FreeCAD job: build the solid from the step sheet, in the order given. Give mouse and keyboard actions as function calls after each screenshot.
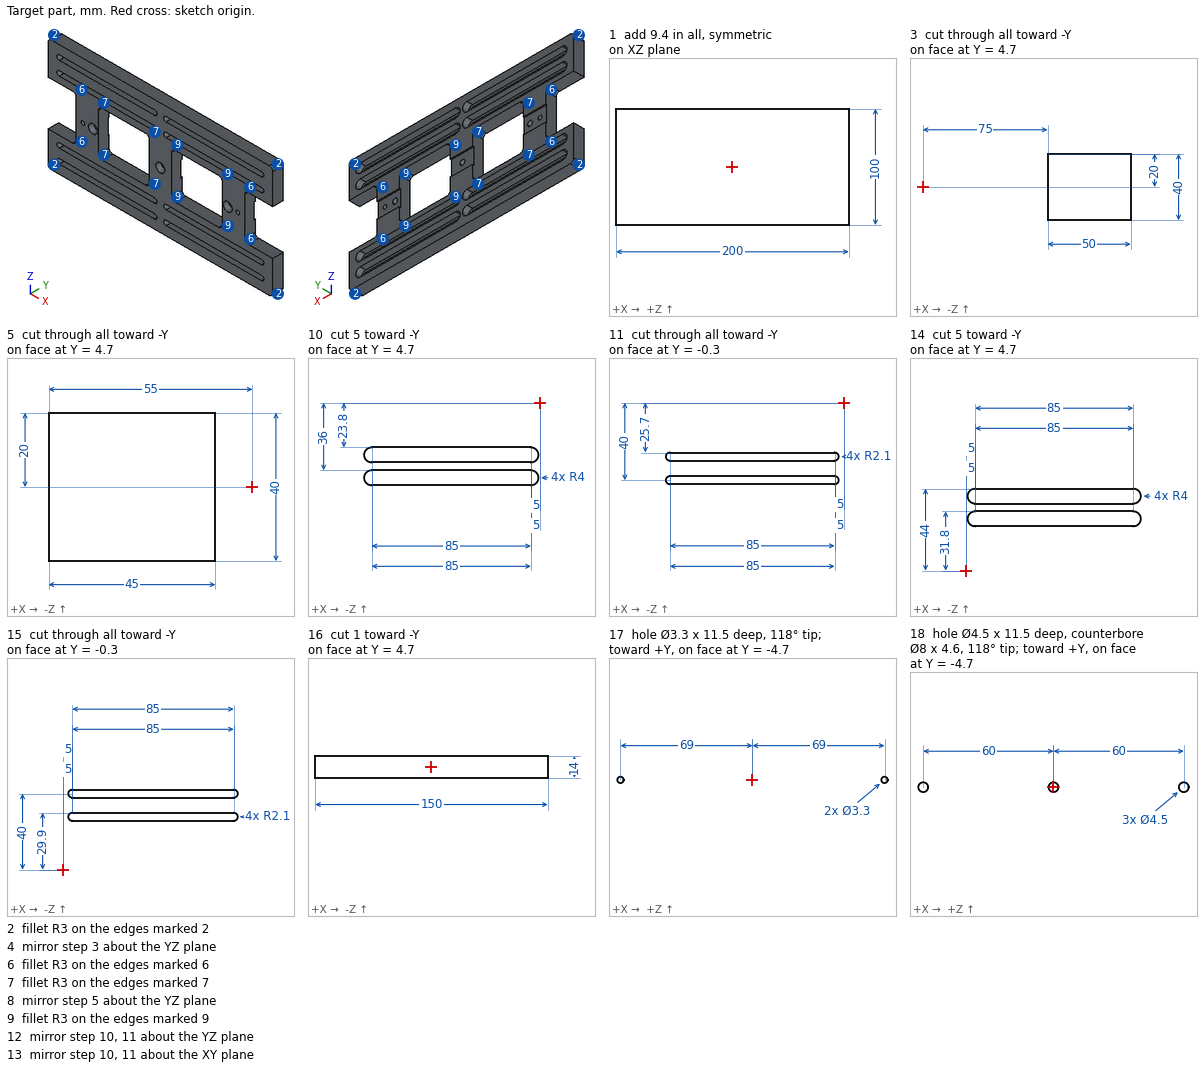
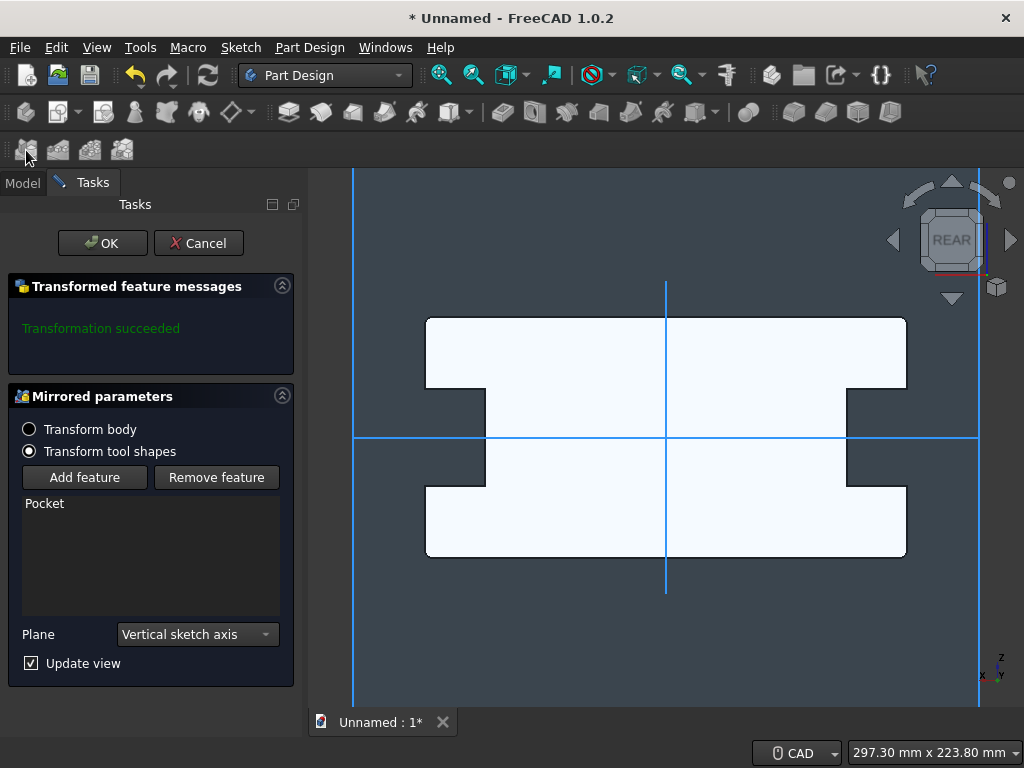
click(198, 634)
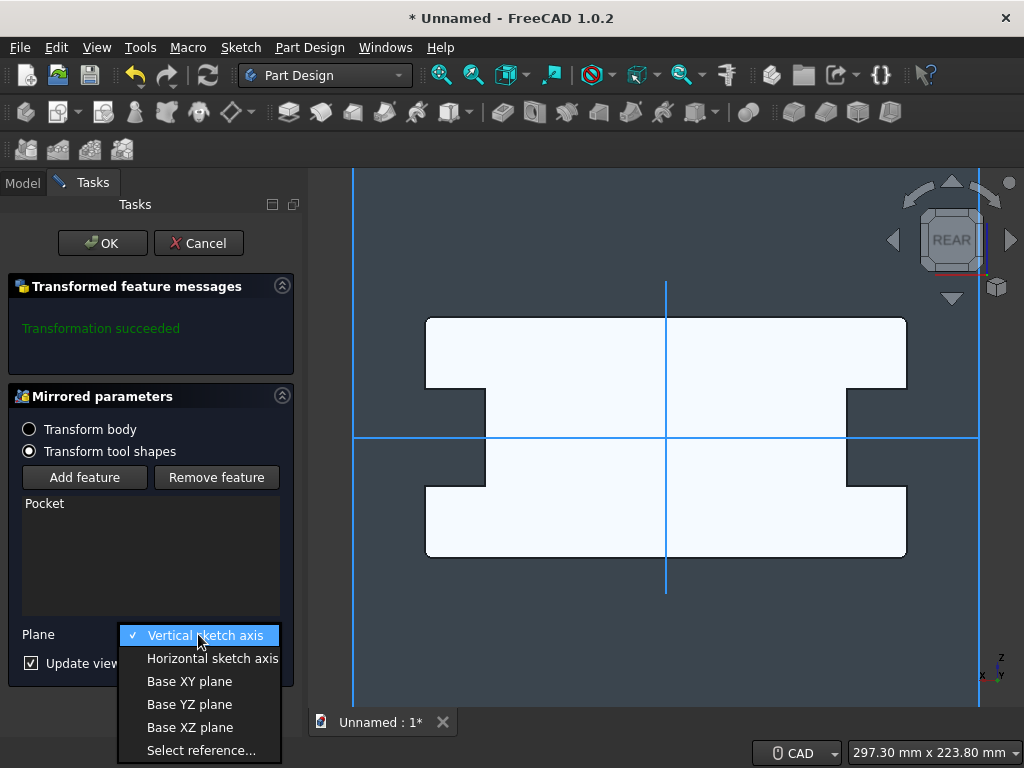
click(198, 704)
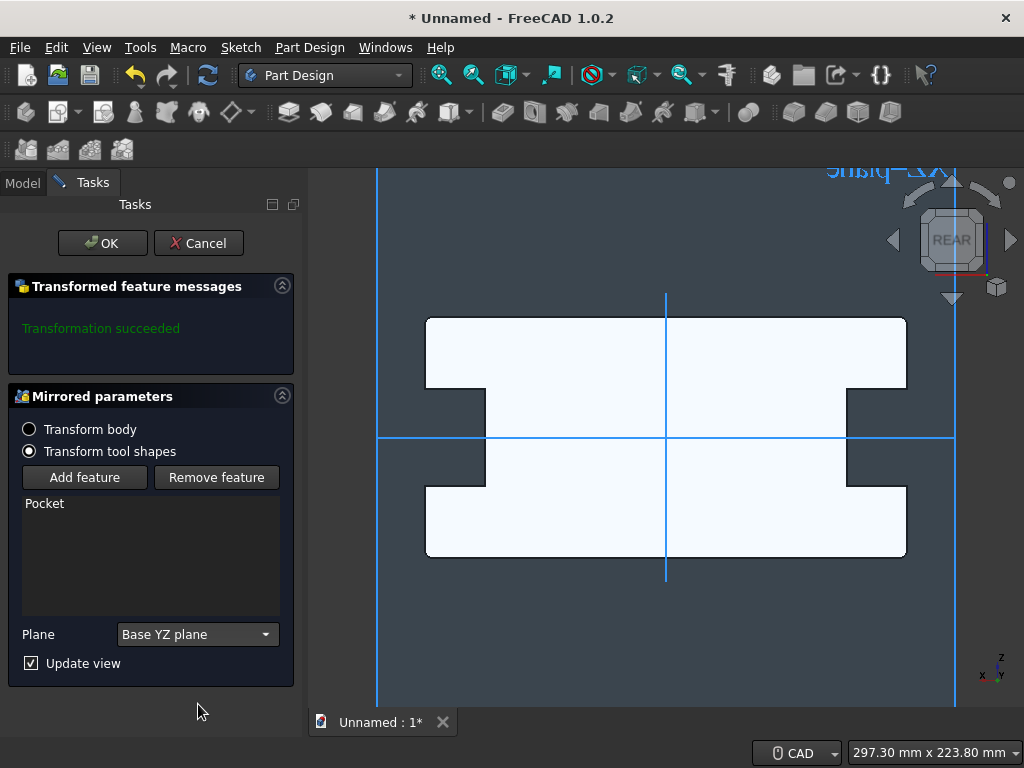
click(103, 243)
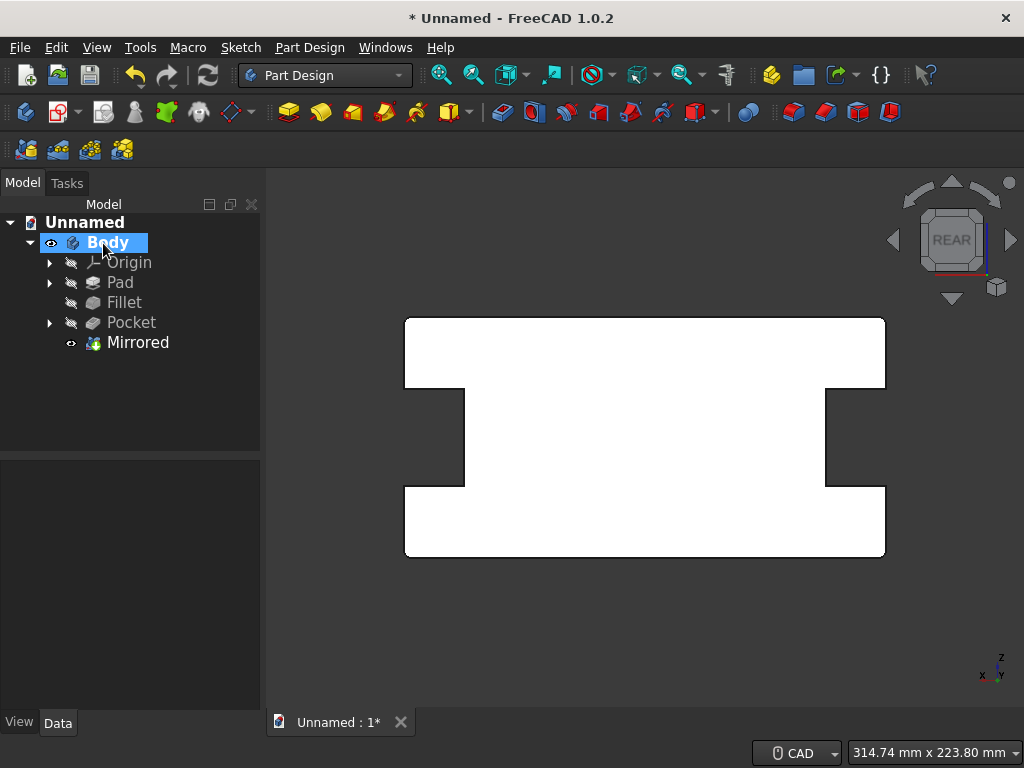
click(645, 437)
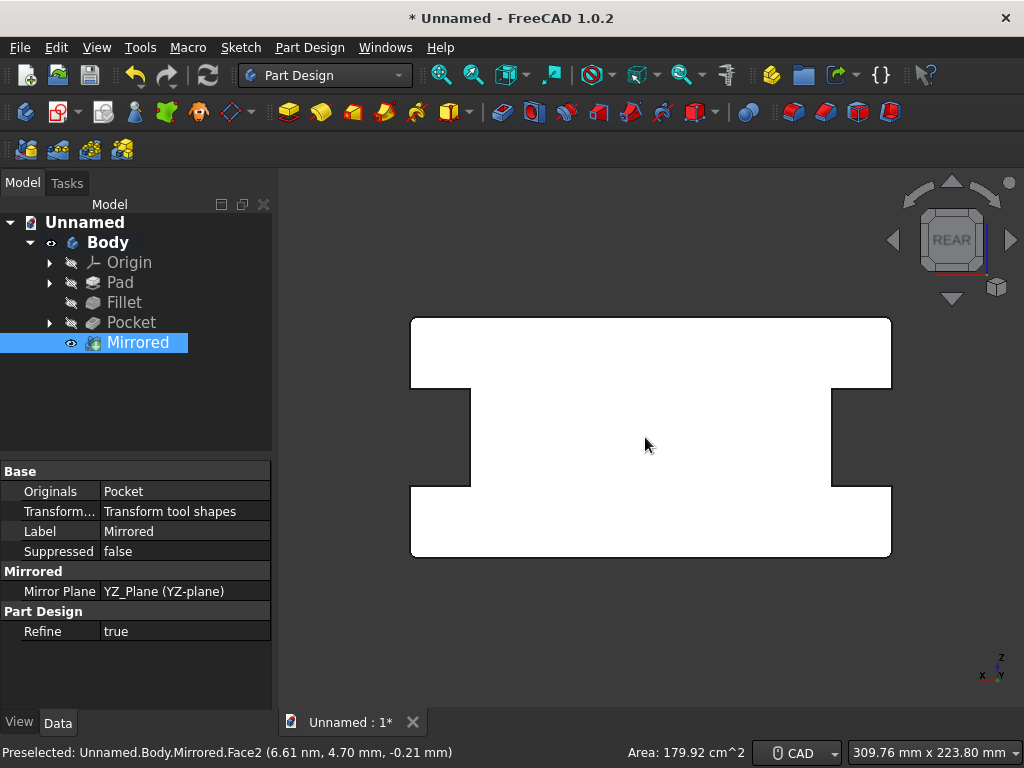
click(58, 112)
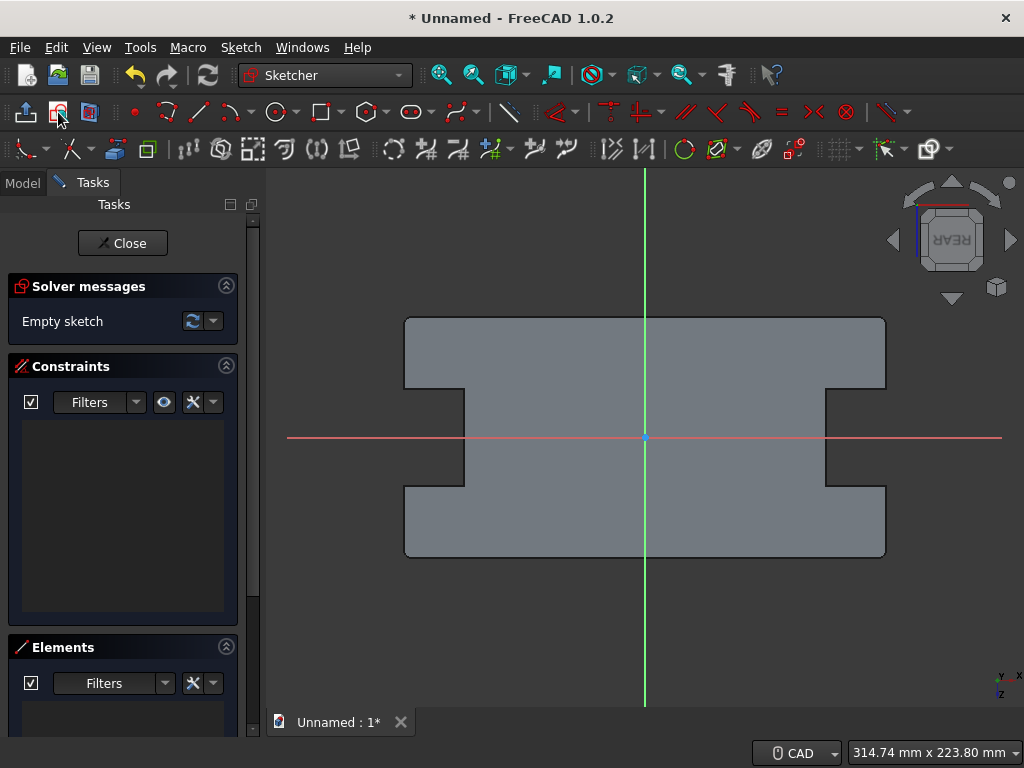
scroll(580, 437, up, 6)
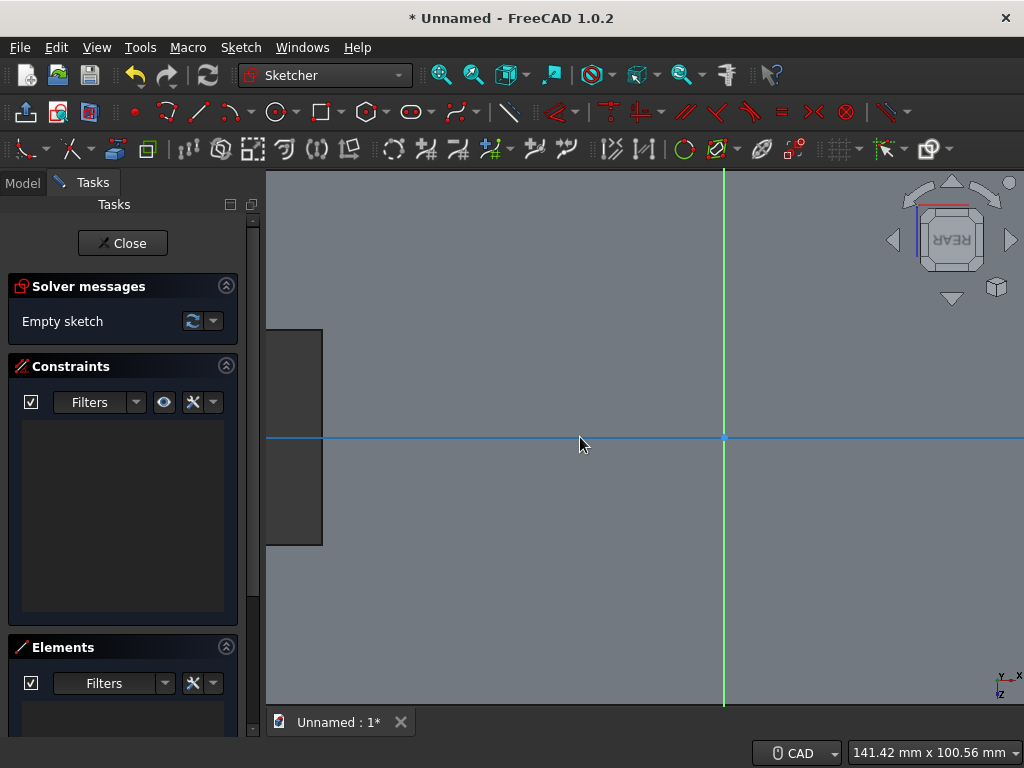
click(322, 112)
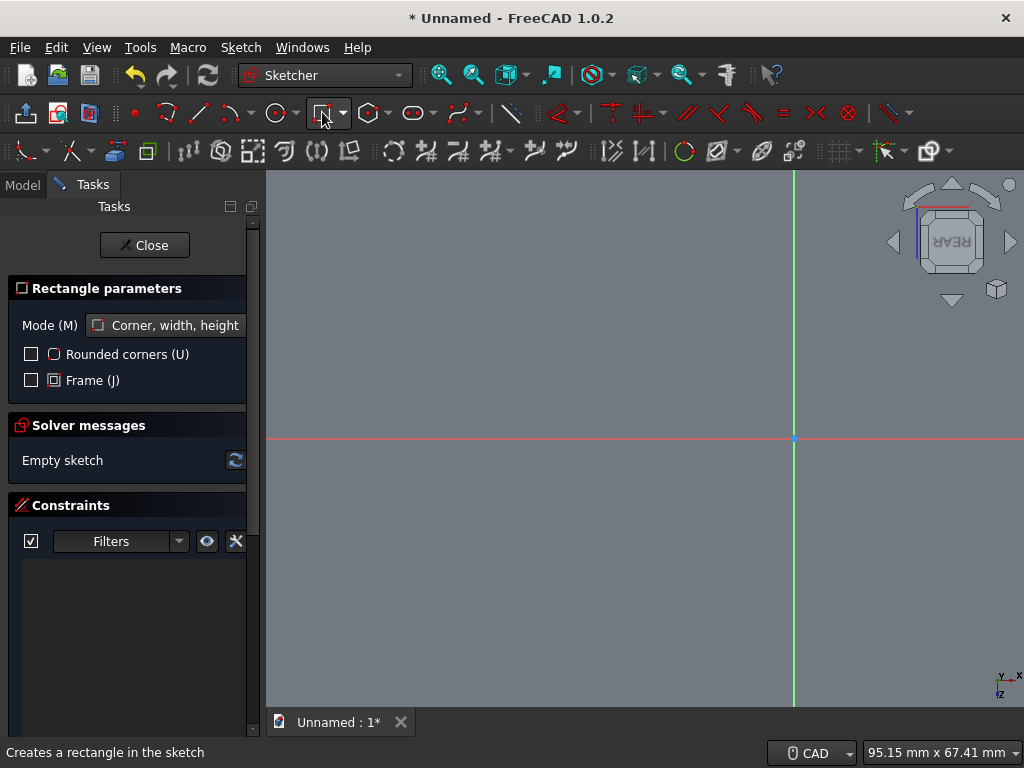
click(356, 279)
move(715, 598)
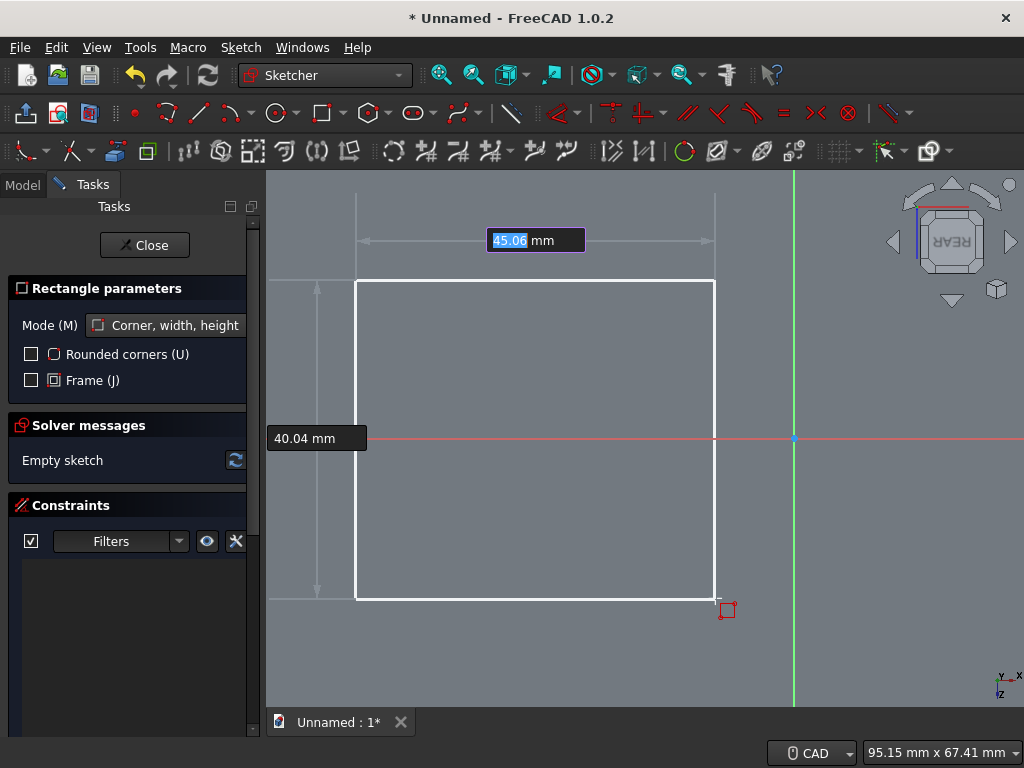
text(45)
key(Tab)
text(40)
key(Return)
key(Escape)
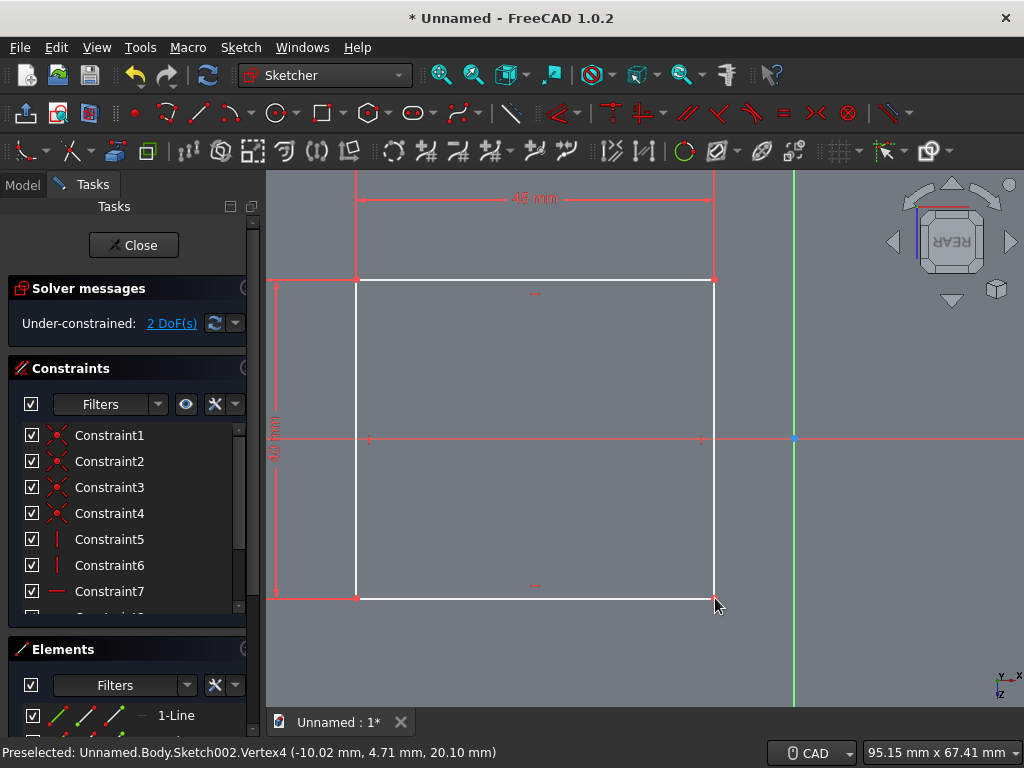
key(d)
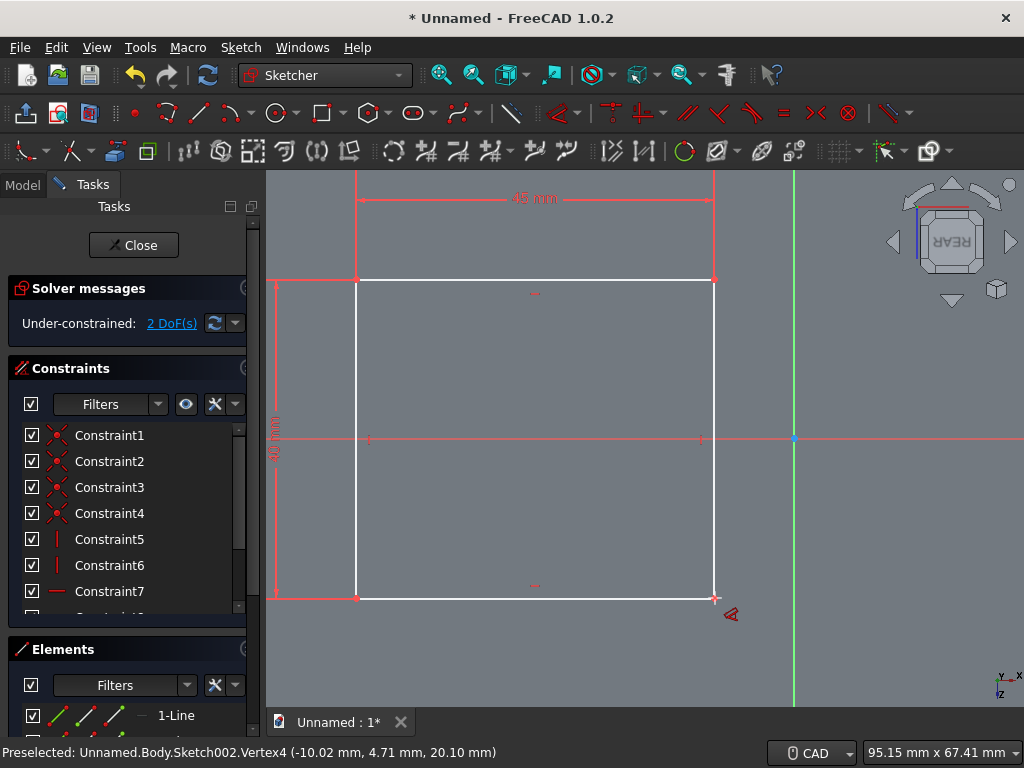
click(356, 280)
click(575, 246)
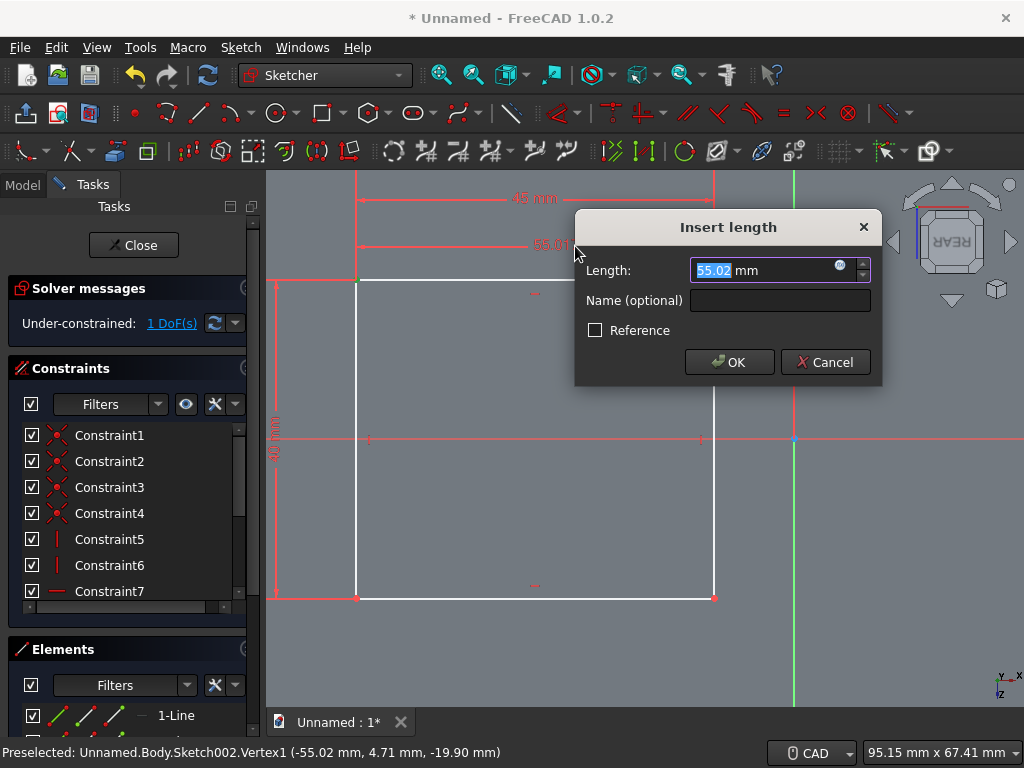
text(55)
key(Return)